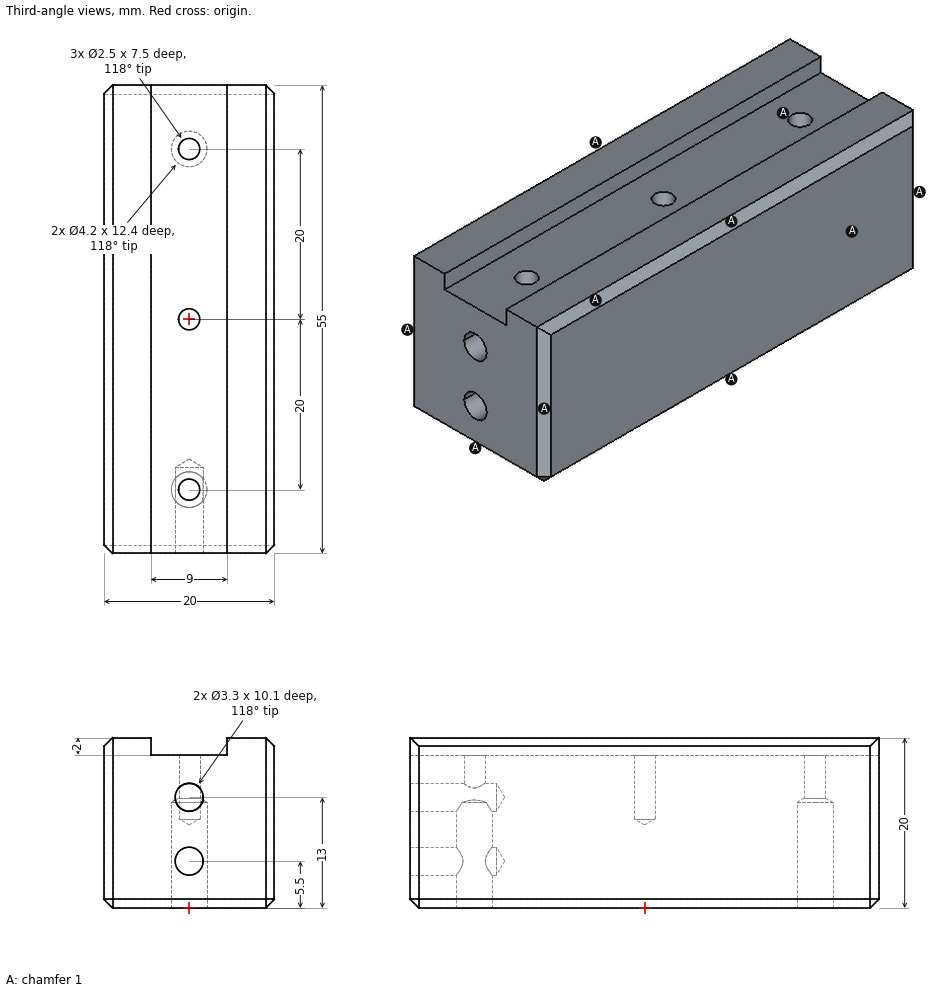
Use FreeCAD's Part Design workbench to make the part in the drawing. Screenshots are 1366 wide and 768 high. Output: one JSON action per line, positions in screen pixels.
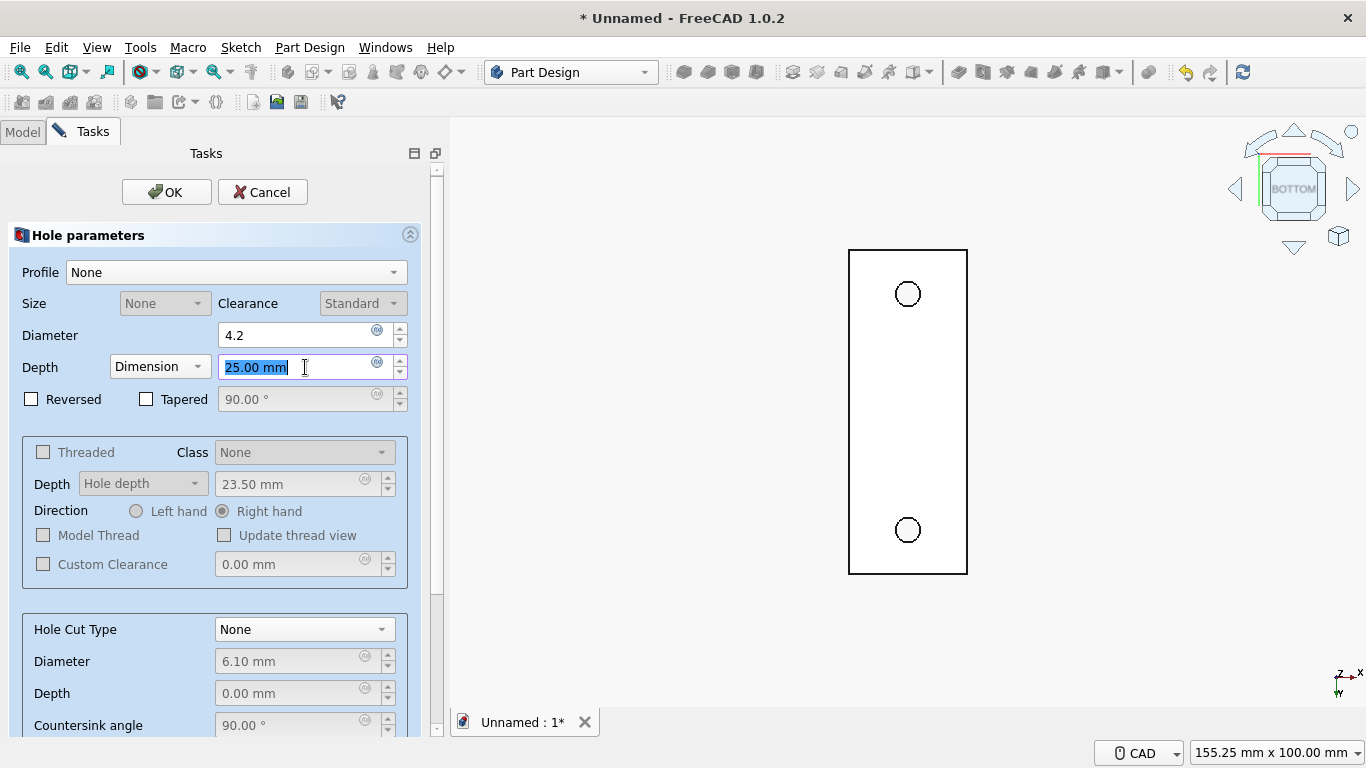
{"action": "type", "text": "12.4"}
{"action": "key", "text": "Tab"}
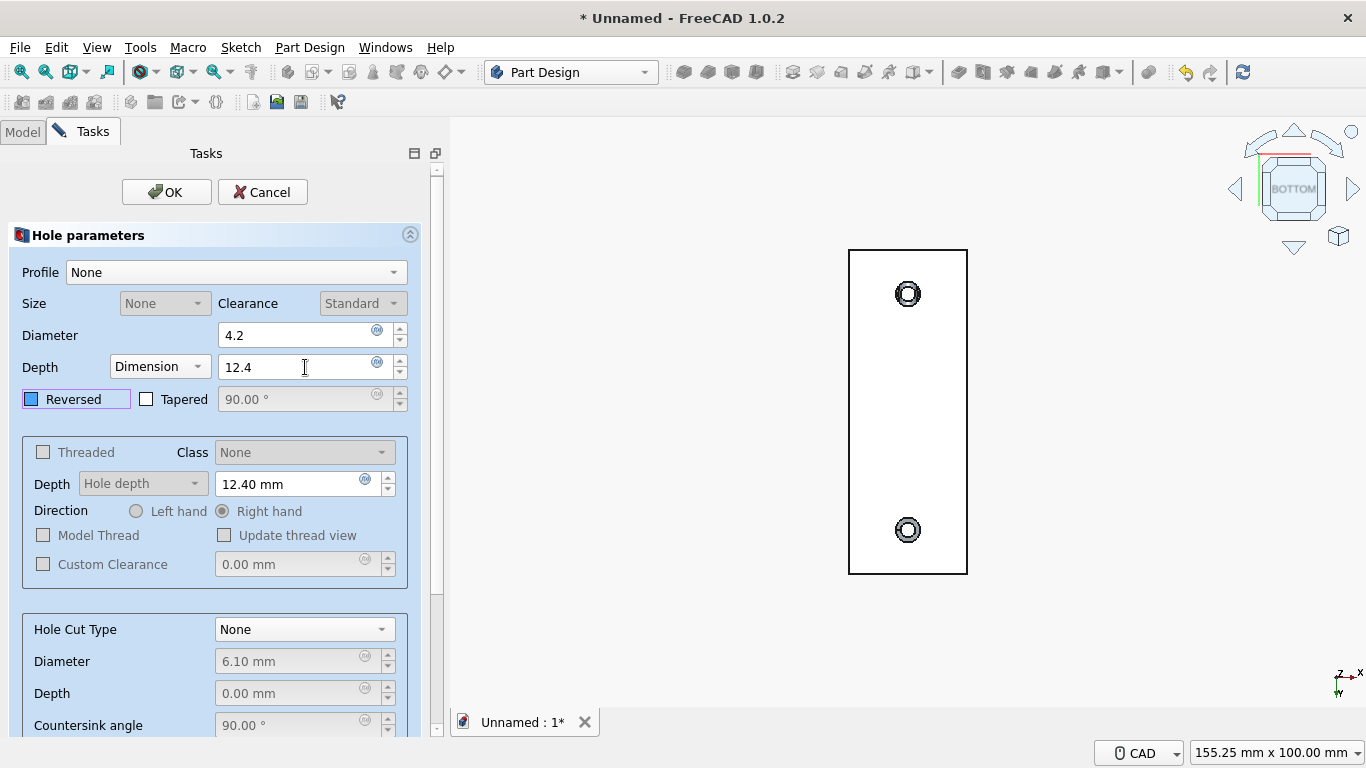
{"action": "left_click", "coordinate": [167, 192]}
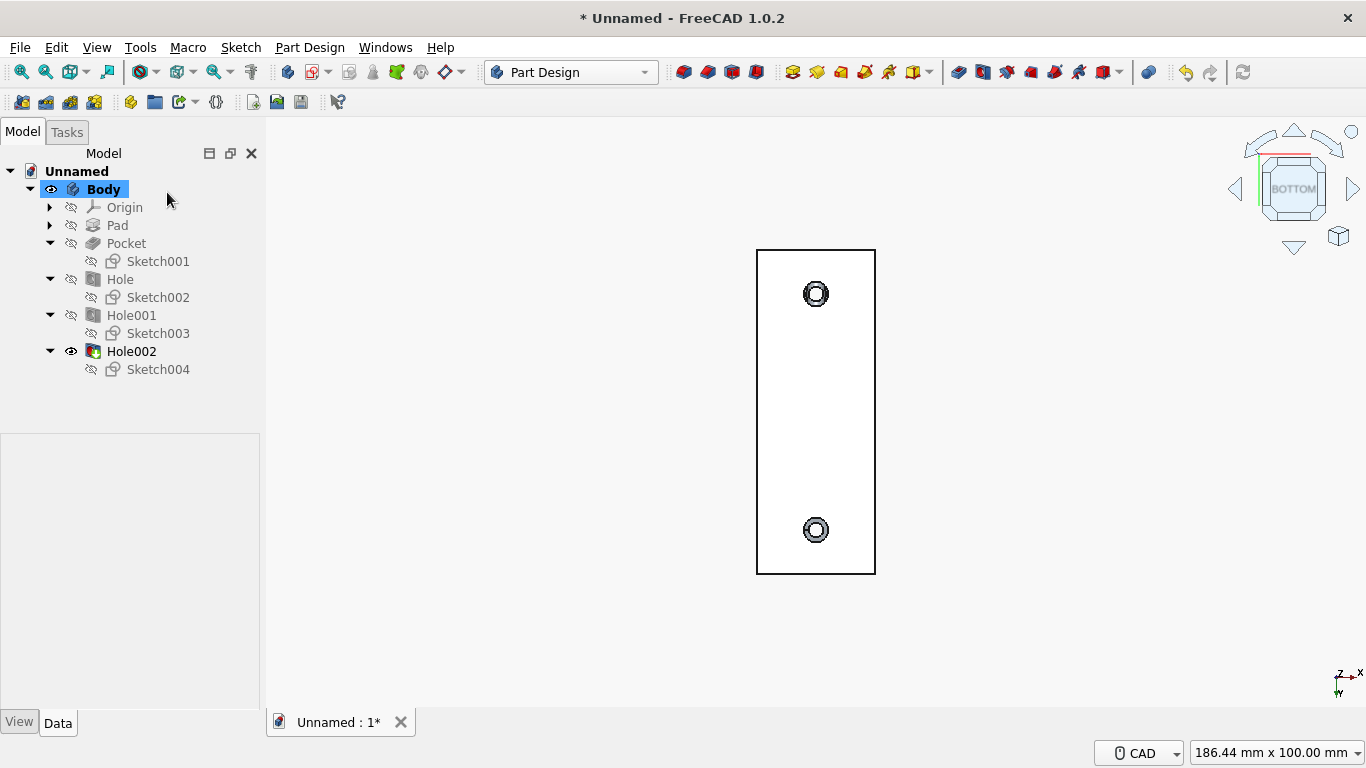
{"action": "left_click", "coordinate": [816, 573]}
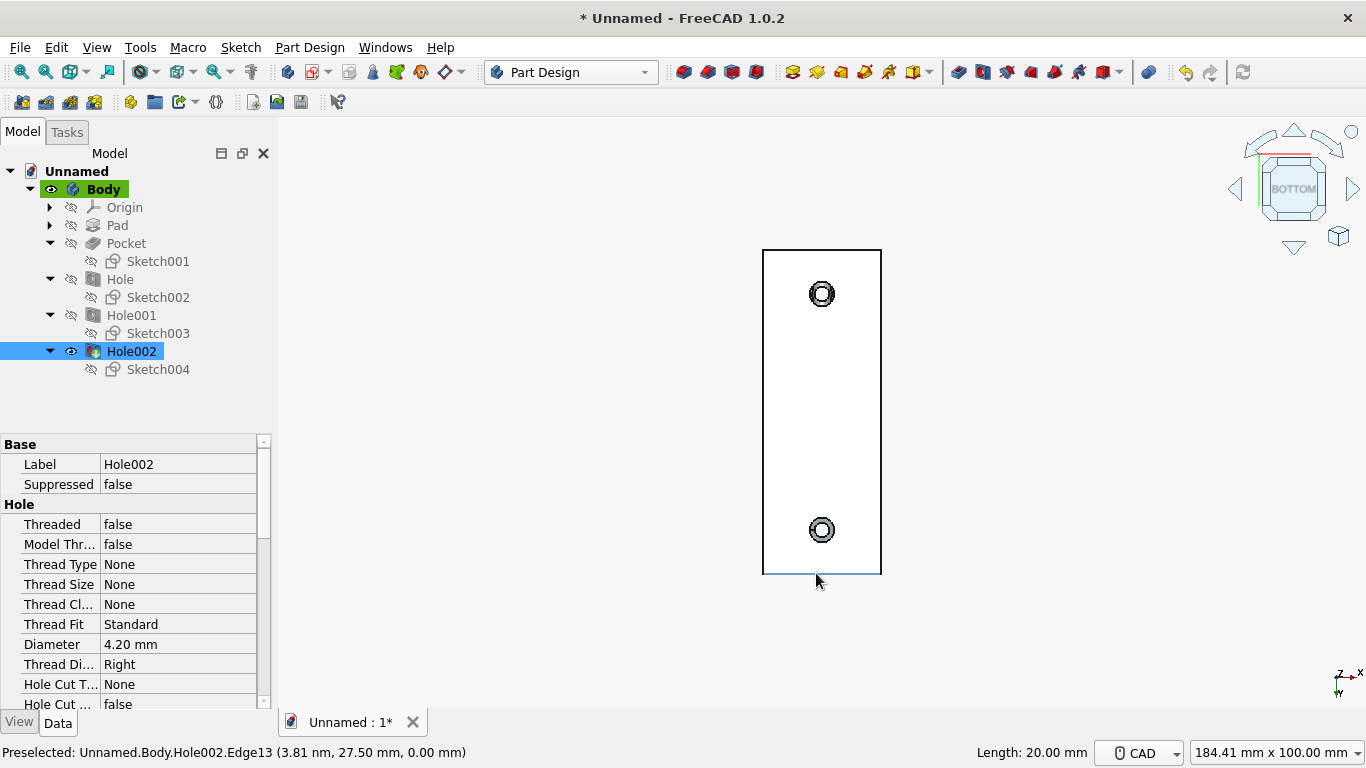
{"action": "key", "text": "0"}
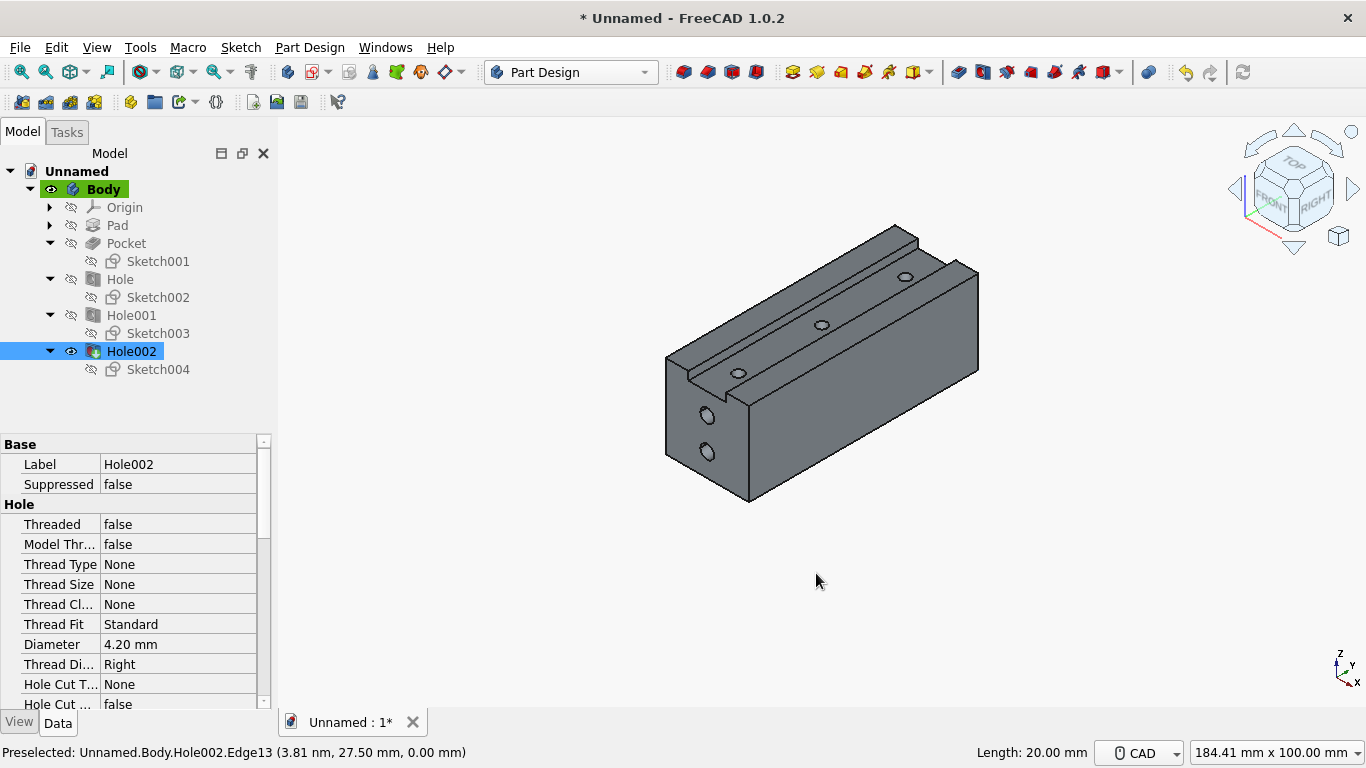
{"action": "left_click", "coordinate": [929, 349], "text": "ctrl"}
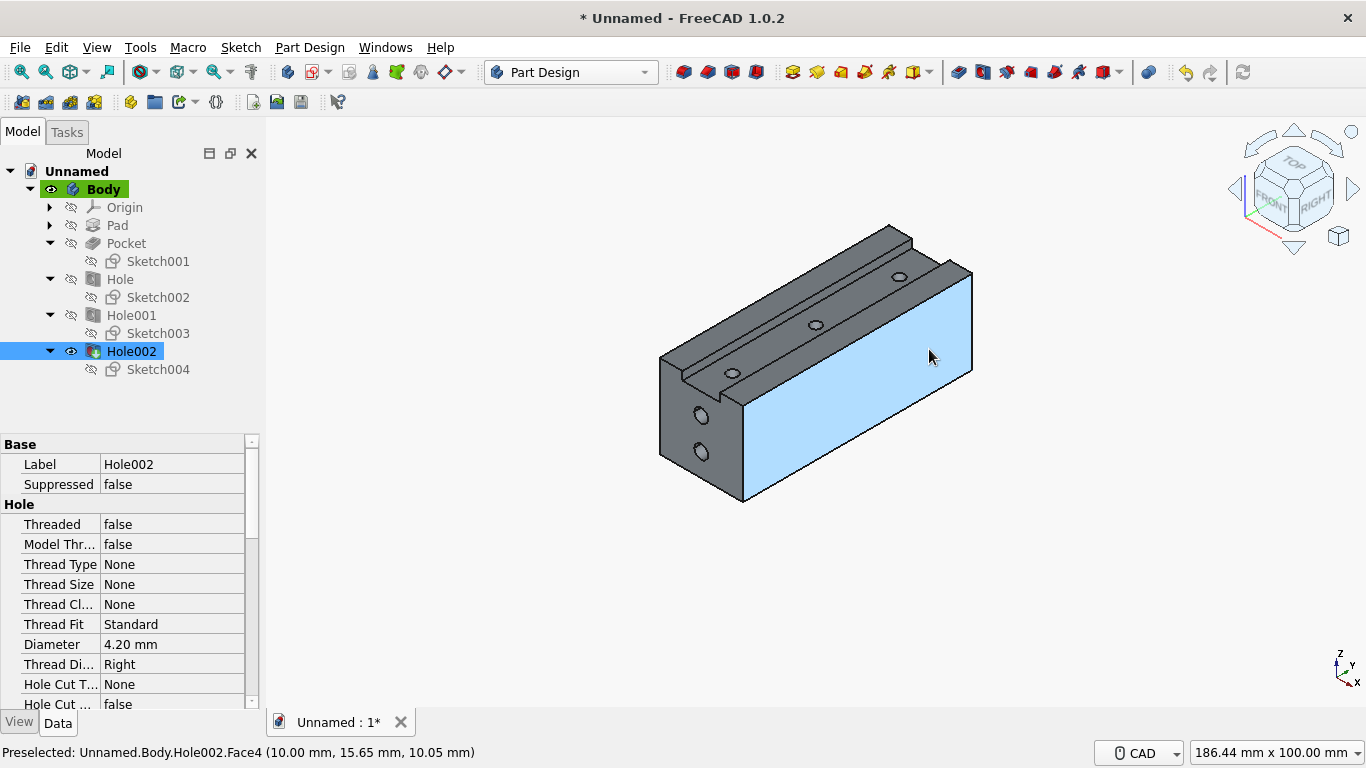
{"action": "key", "text": "2"}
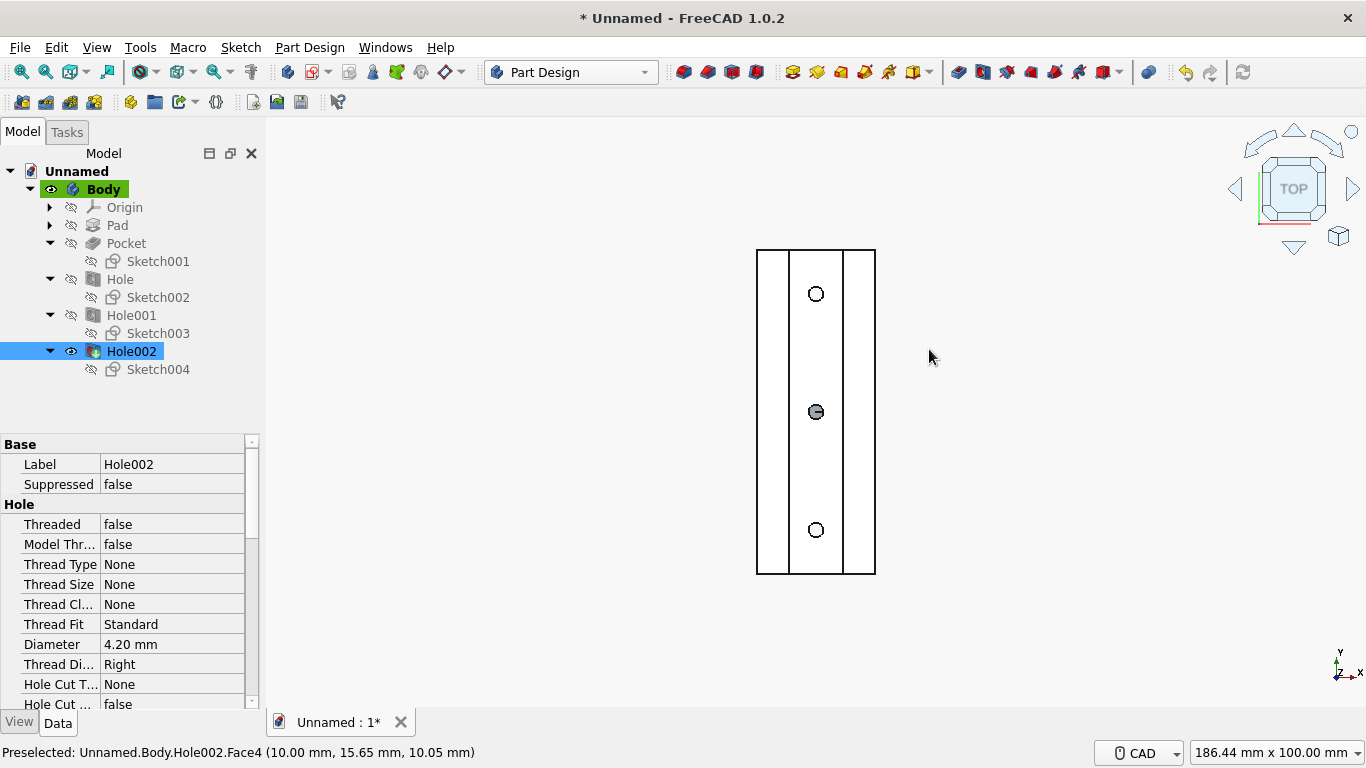
{"action": "key", "text": "1"}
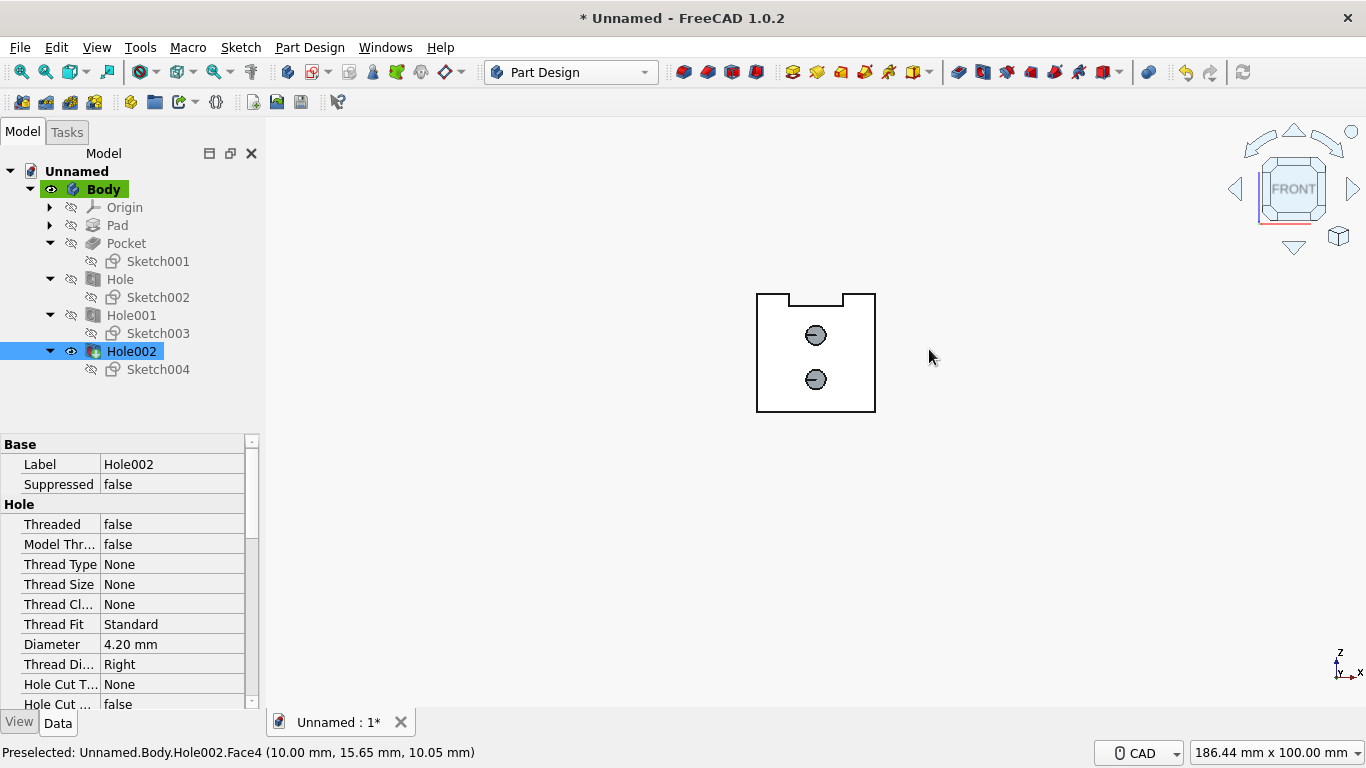
{"action": "left_click", "coordinate": [22, 72]}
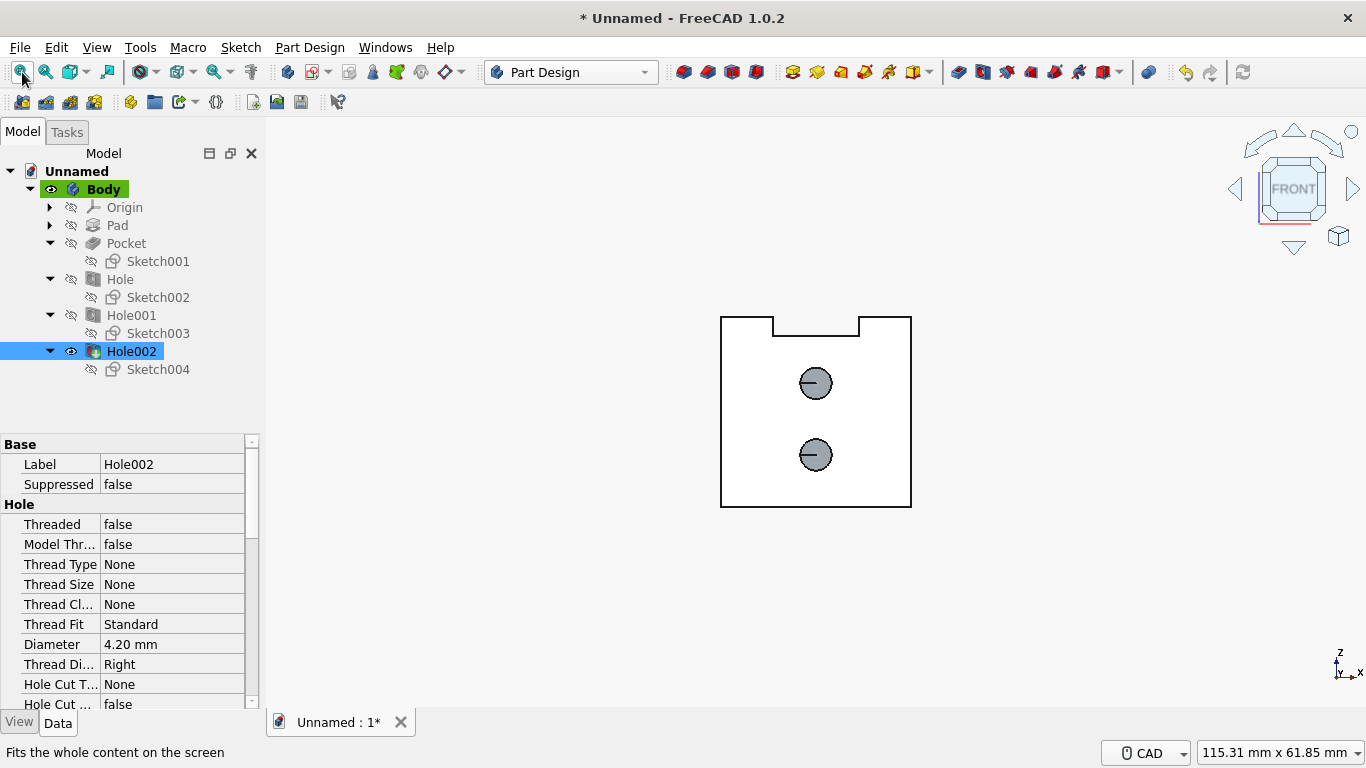
{"action": "left_click", "coordinate": [816, 506], "text": "ctrl"}